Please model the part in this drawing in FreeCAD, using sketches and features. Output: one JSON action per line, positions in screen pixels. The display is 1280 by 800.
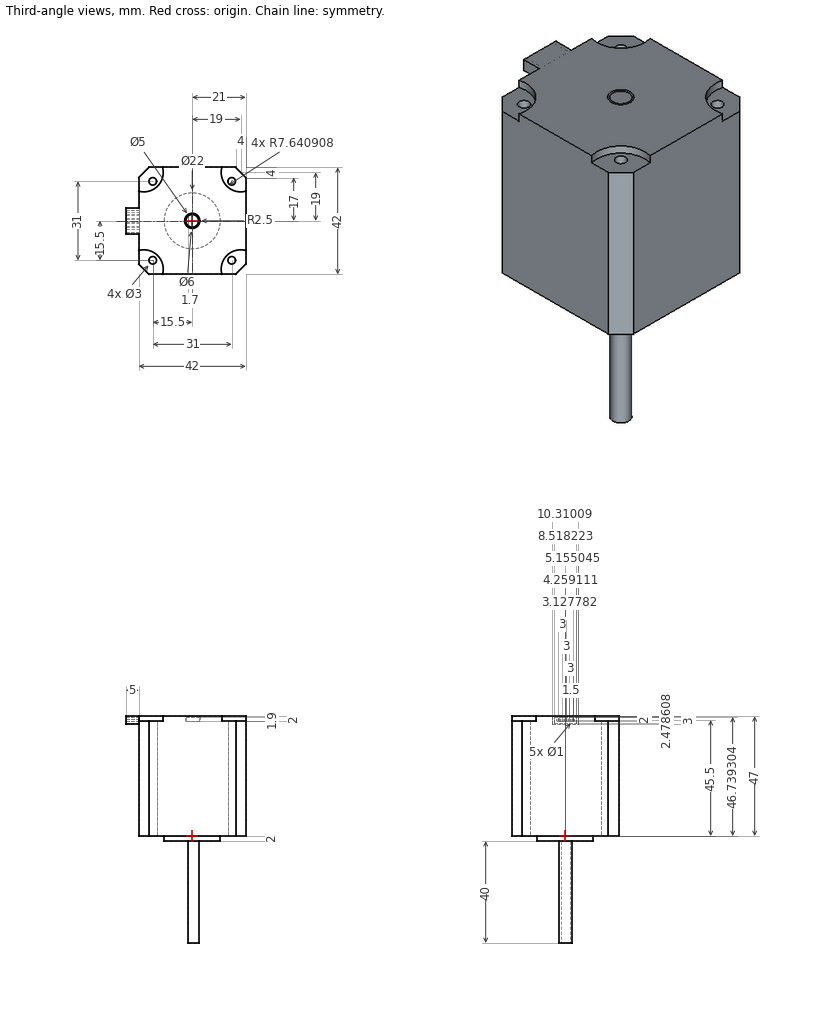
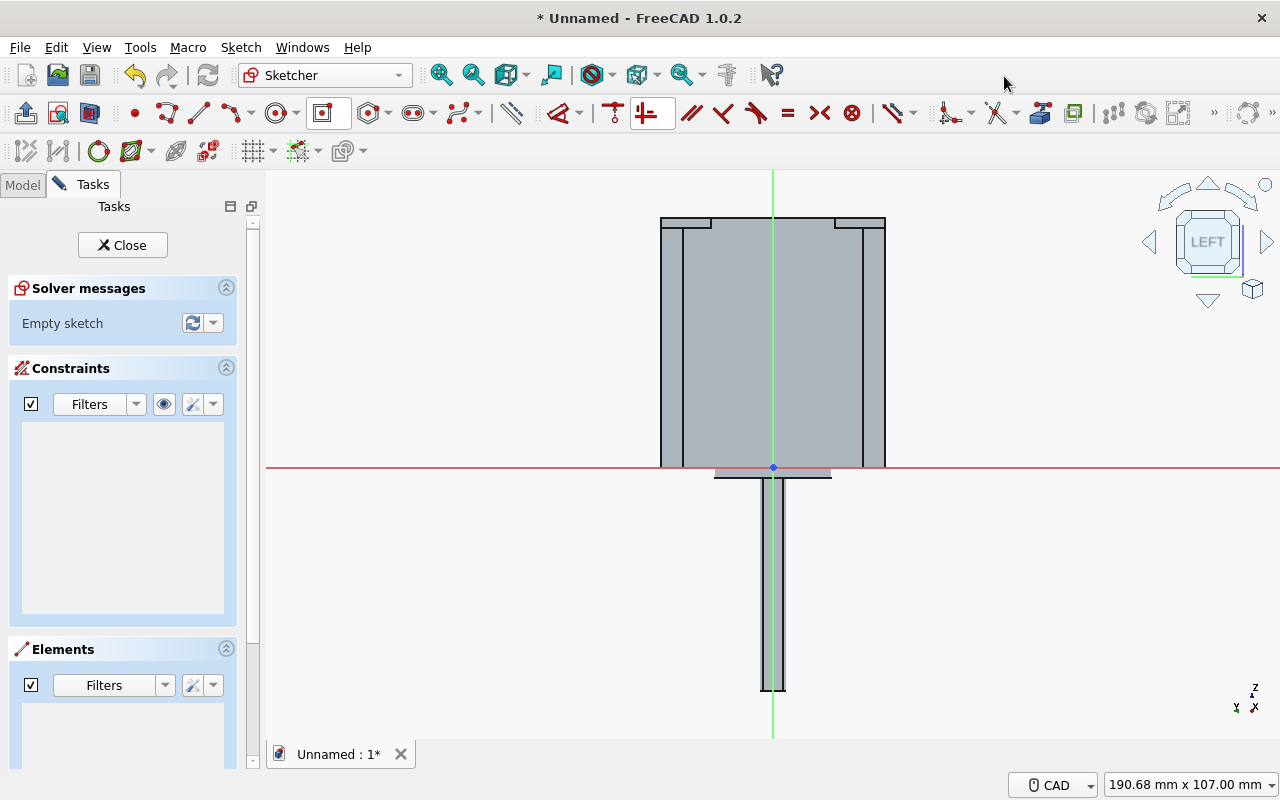
{"action": "scroll", "coordinate": [780, 203], "scroll_direction": "up", "scroll_amount": 12}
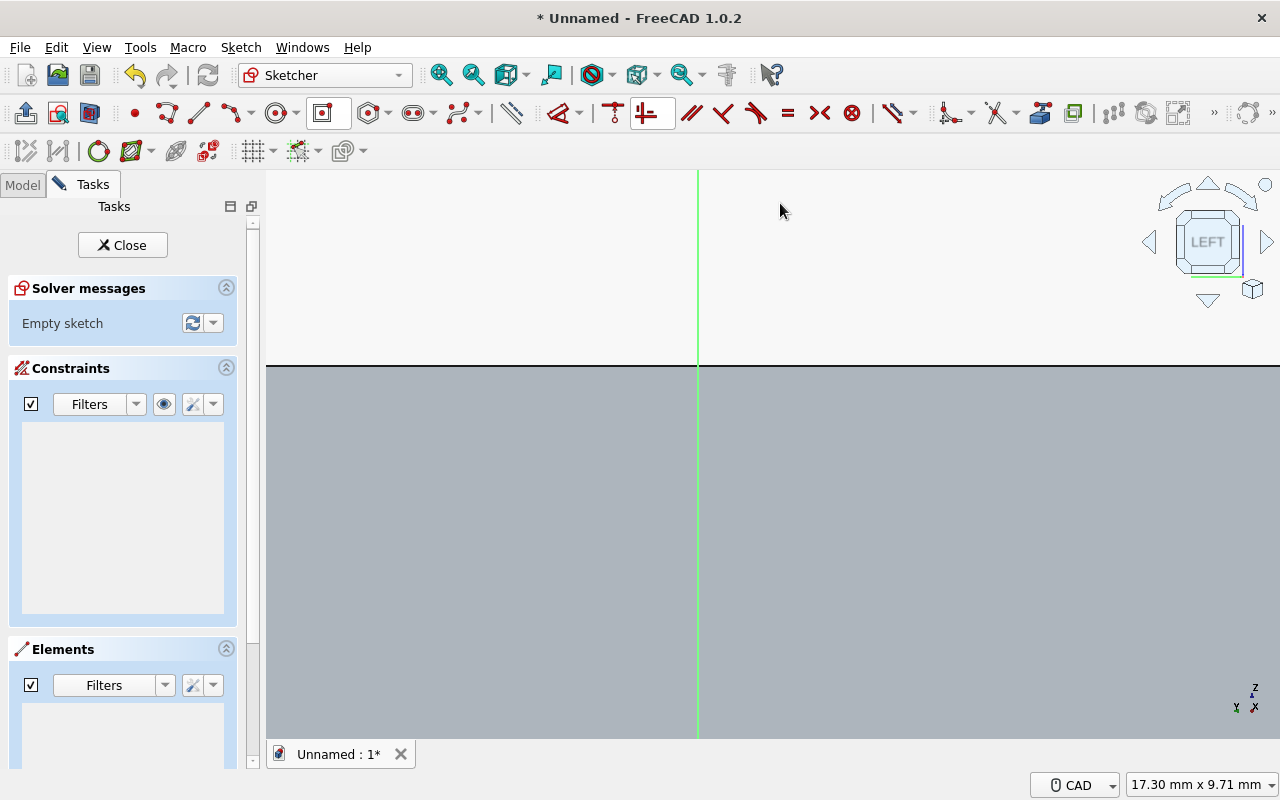
{"action": "key", "text": "g r"}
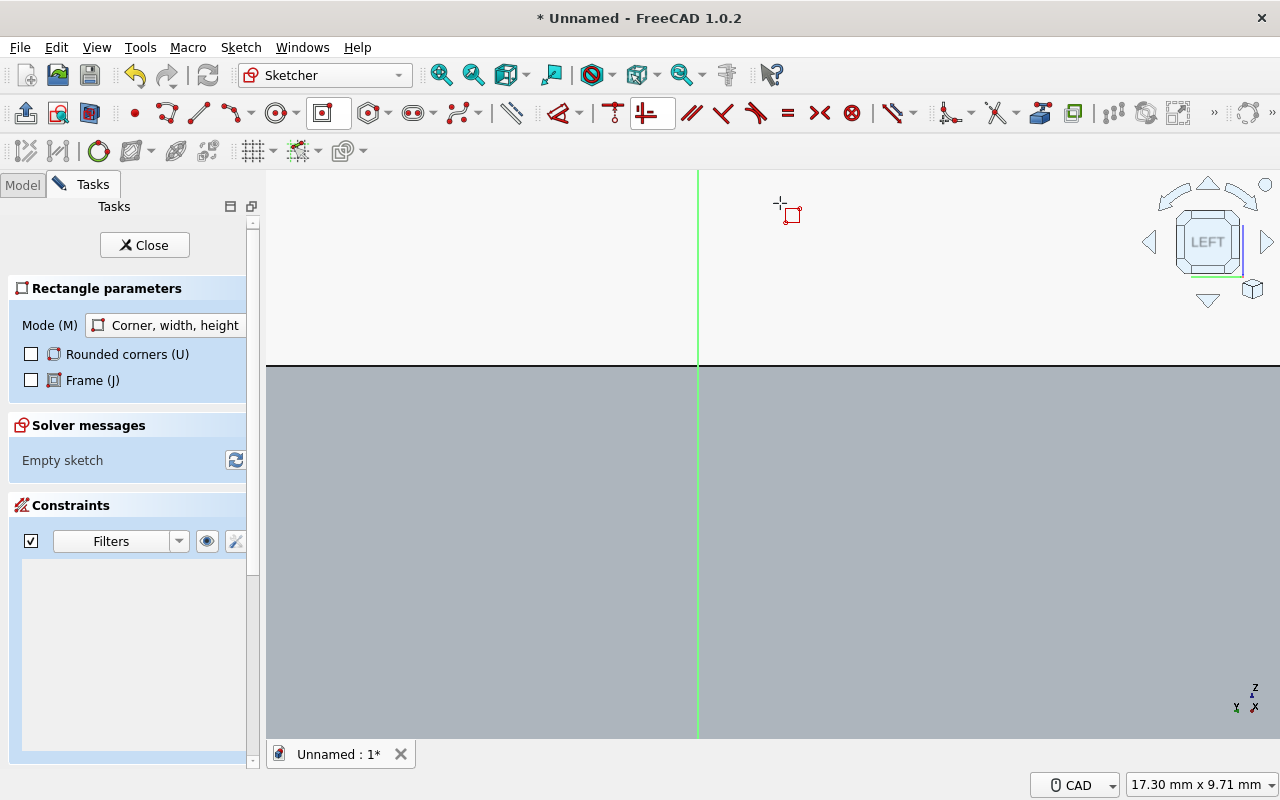
{"action": "left_click", "coordinate": [396, 366]}
{"action": "left_click", "coordinate": [1000, 542]}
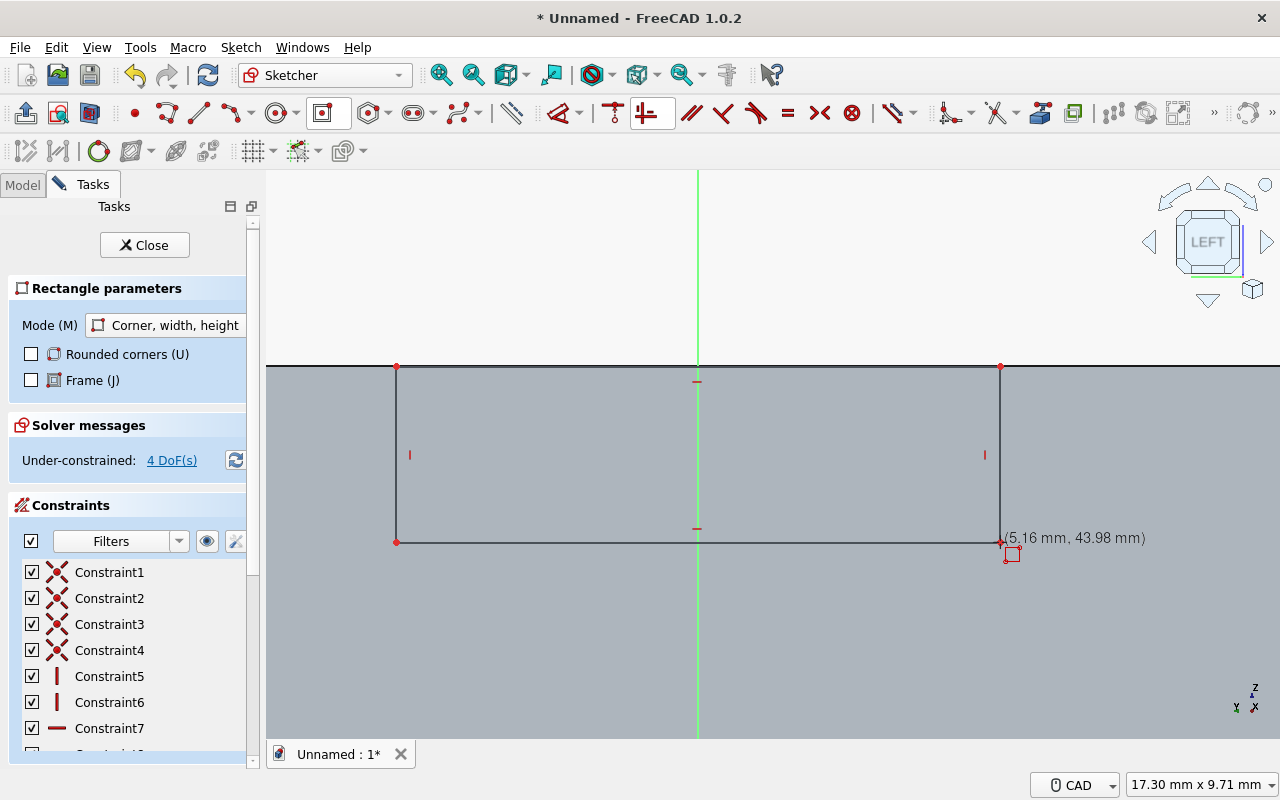
{"action": "left_click", "coordinate": [448, 382]}
{"action": "left_click", "coordinate": [947, 527]}
{"action": "key", "text": "Escape"}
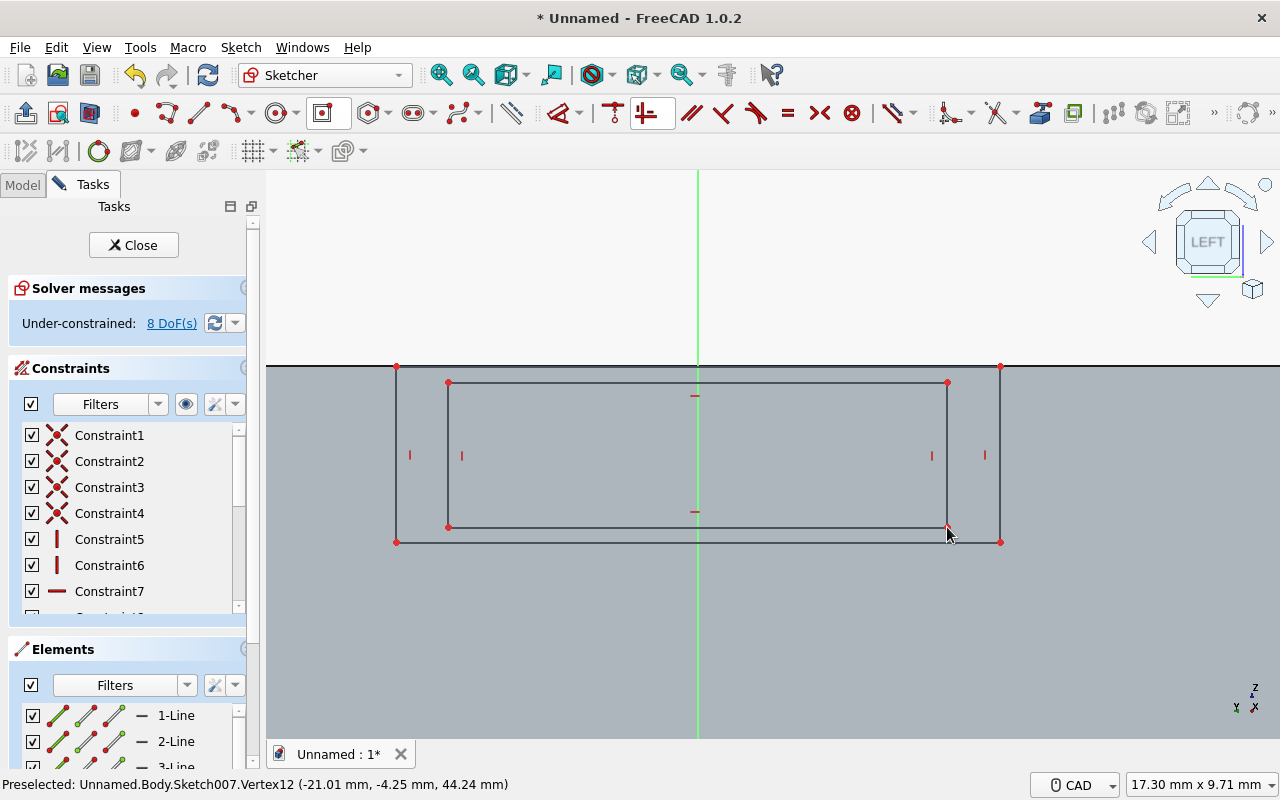
{"action": "left_click", "coordinate": [558, 114]}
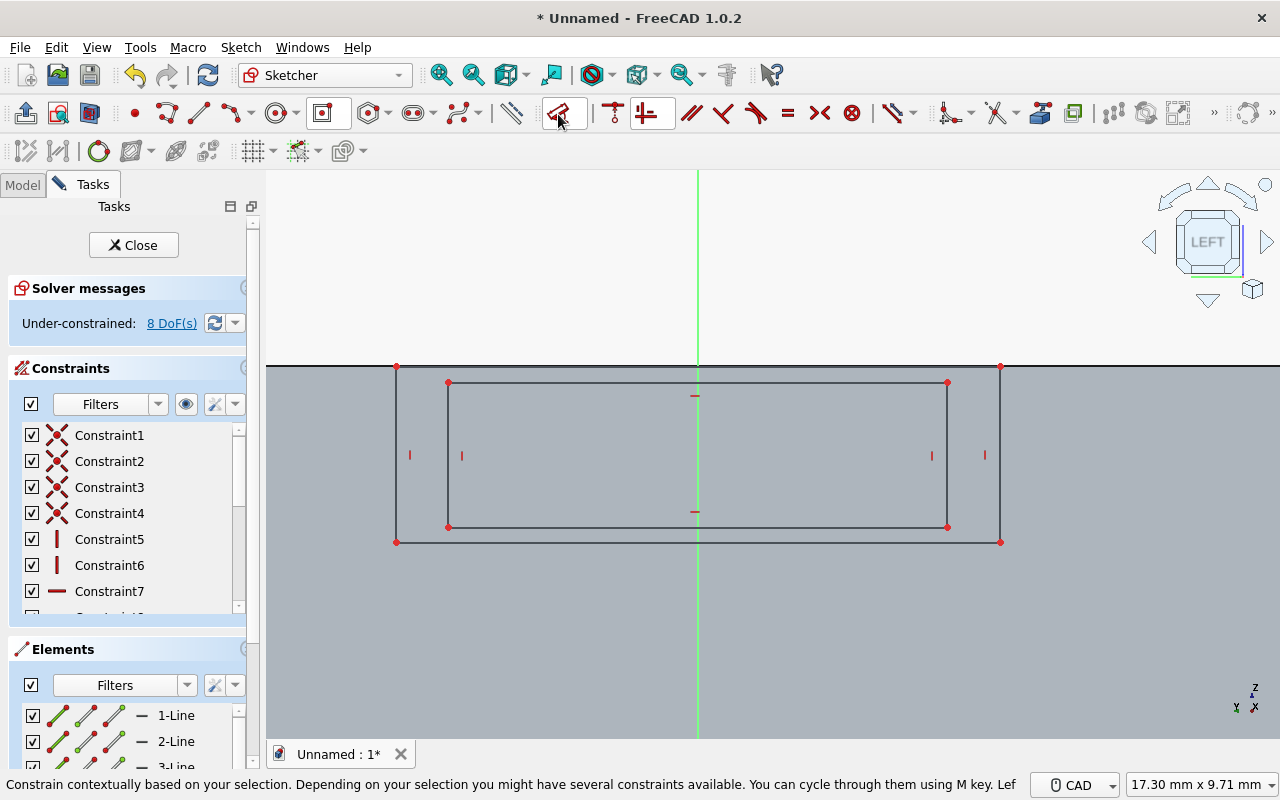
{"action": "left_click", "coordinate": [396, 420]}
{"action": "left_click", "coordinate": [362, 455]}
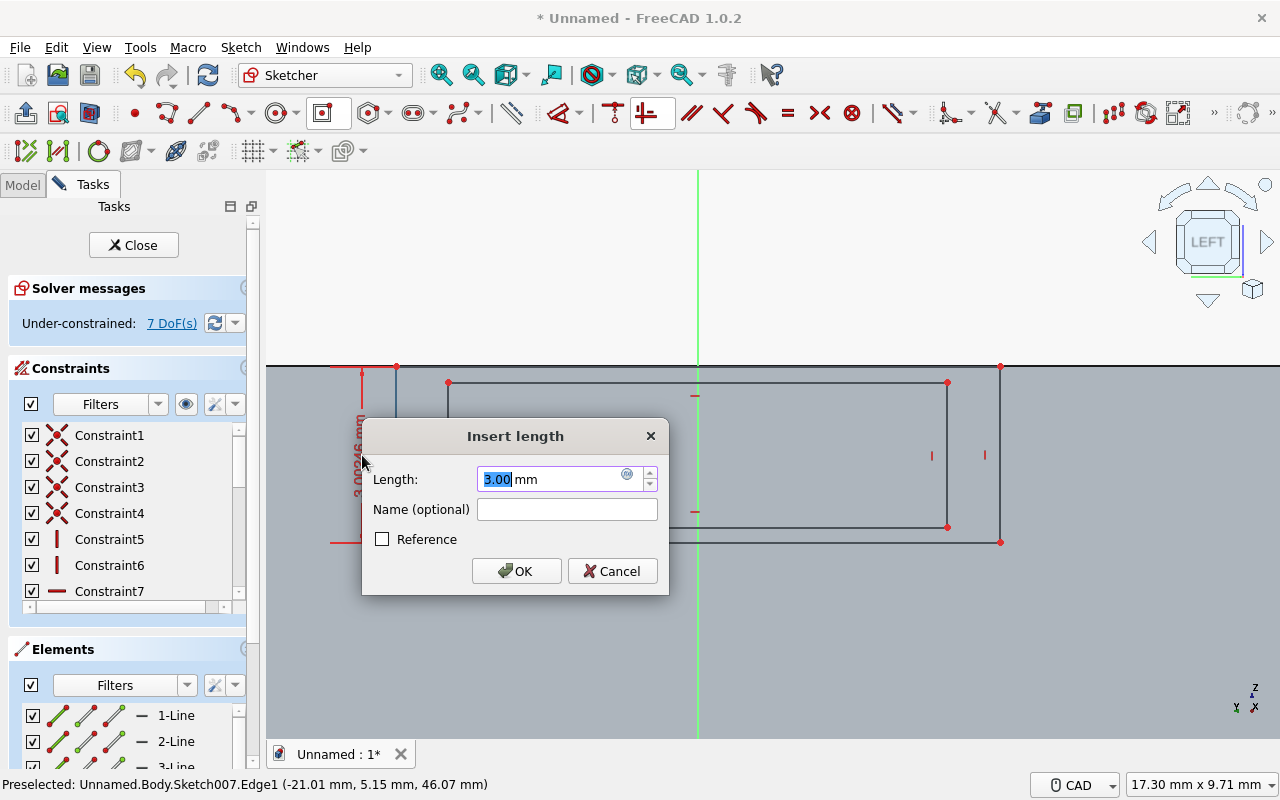
{"action": "type", "text": "3"}
{"action": "key", "text": "Return"}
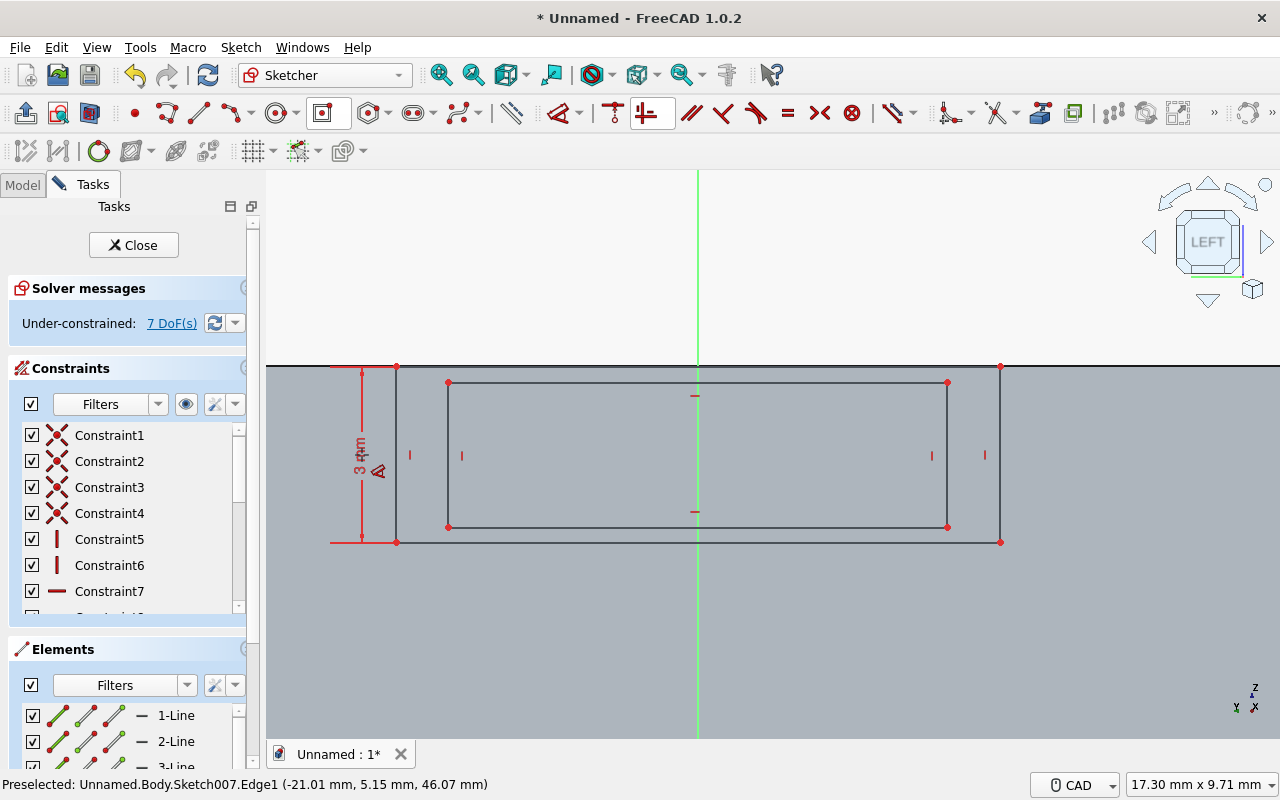
{"action": "left_click", "coordinate": [396, 367]}
{"action": "left_click", "coordinate": [362, 539]}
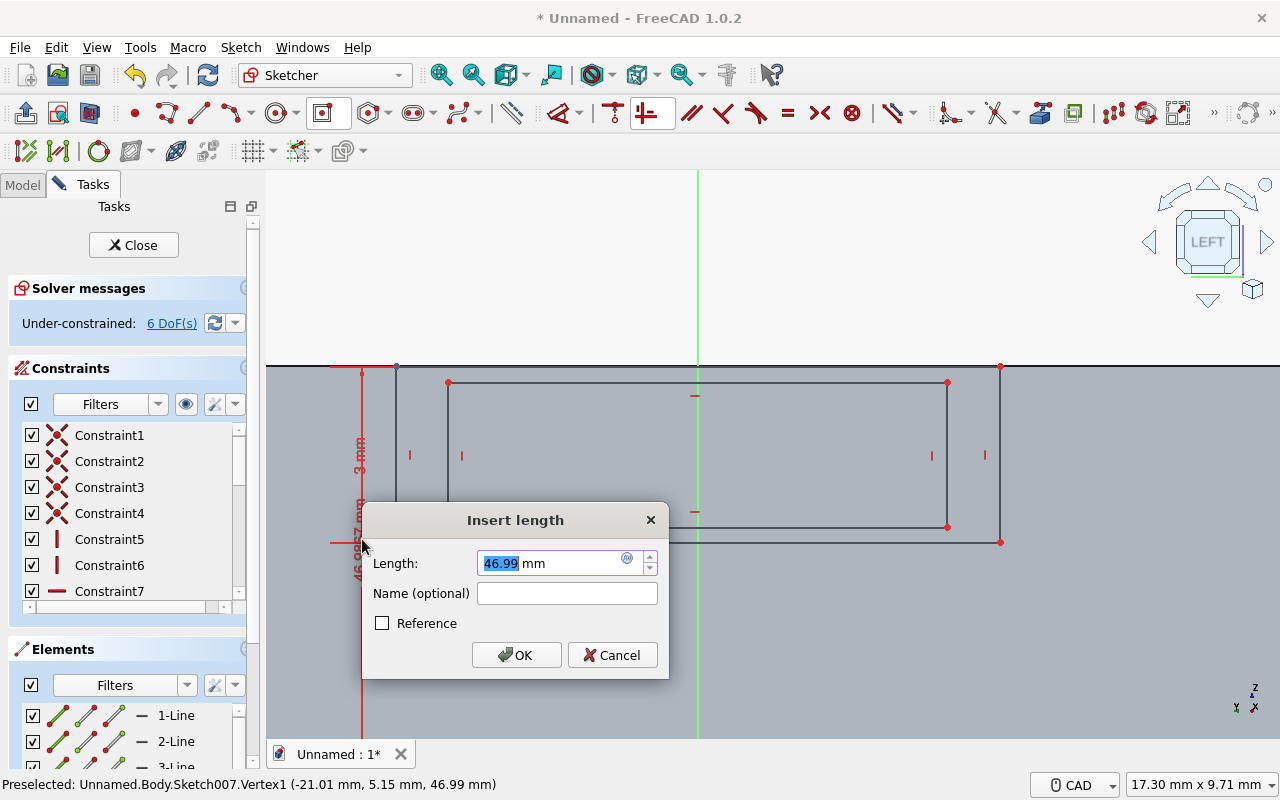
{"action": "type", "text": "47"}
{"action": "key", "text": "Return"}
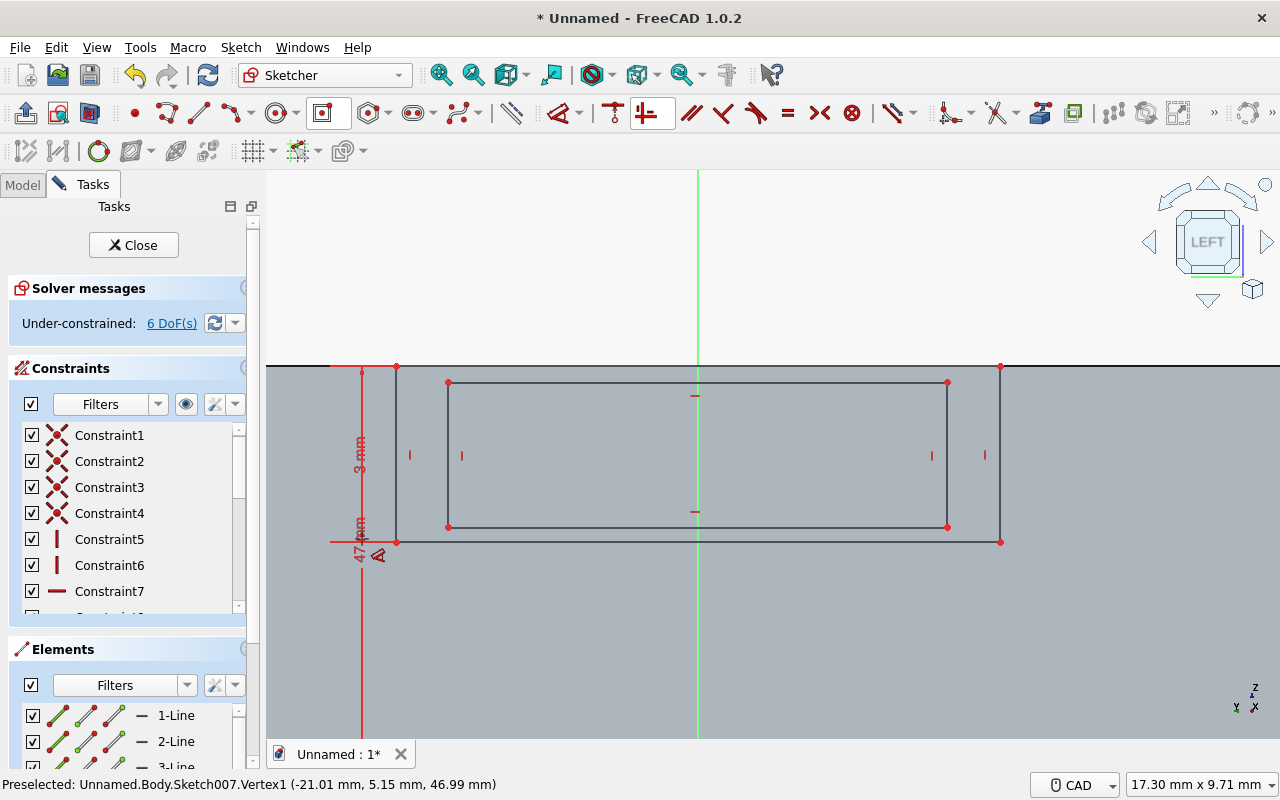
{"action": "left_click", "coordinate": [577, 542]}
{"action": "left_click", "coordinate": [559, 576]}